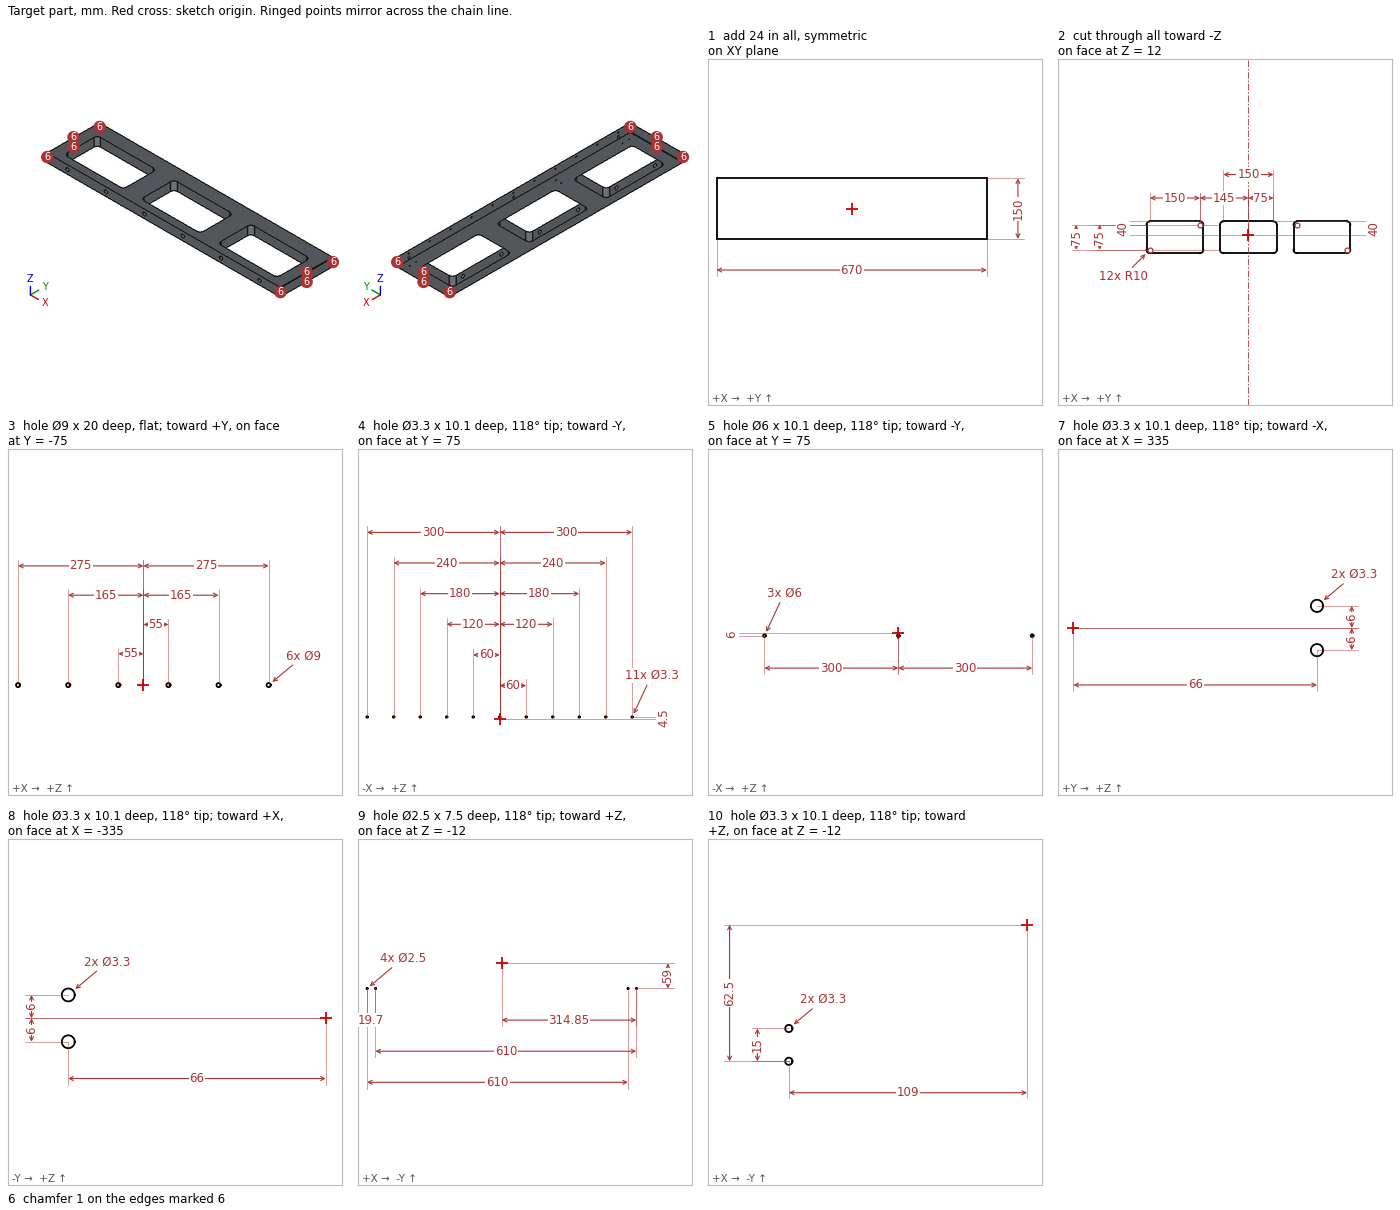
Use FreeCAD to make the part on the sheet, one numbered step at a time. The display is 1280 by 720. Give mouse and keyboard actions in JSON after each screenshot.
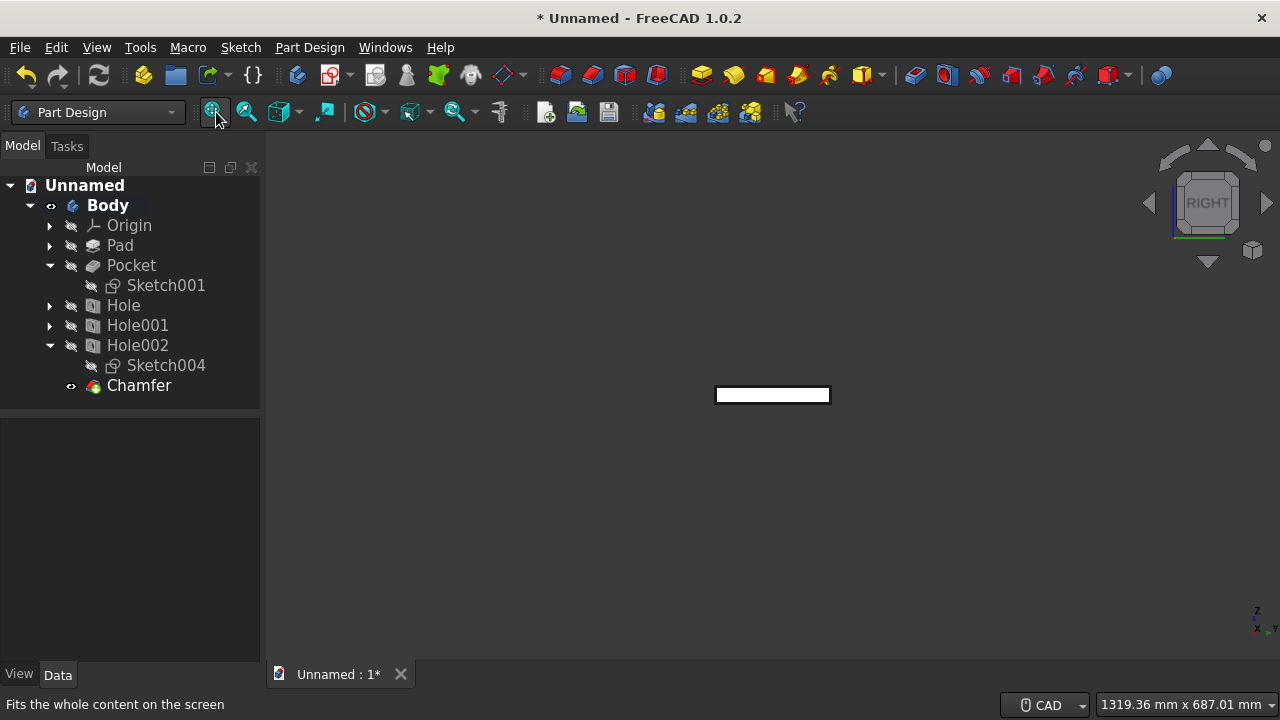
{"action": "left_click", "coordinate": [805, 394]}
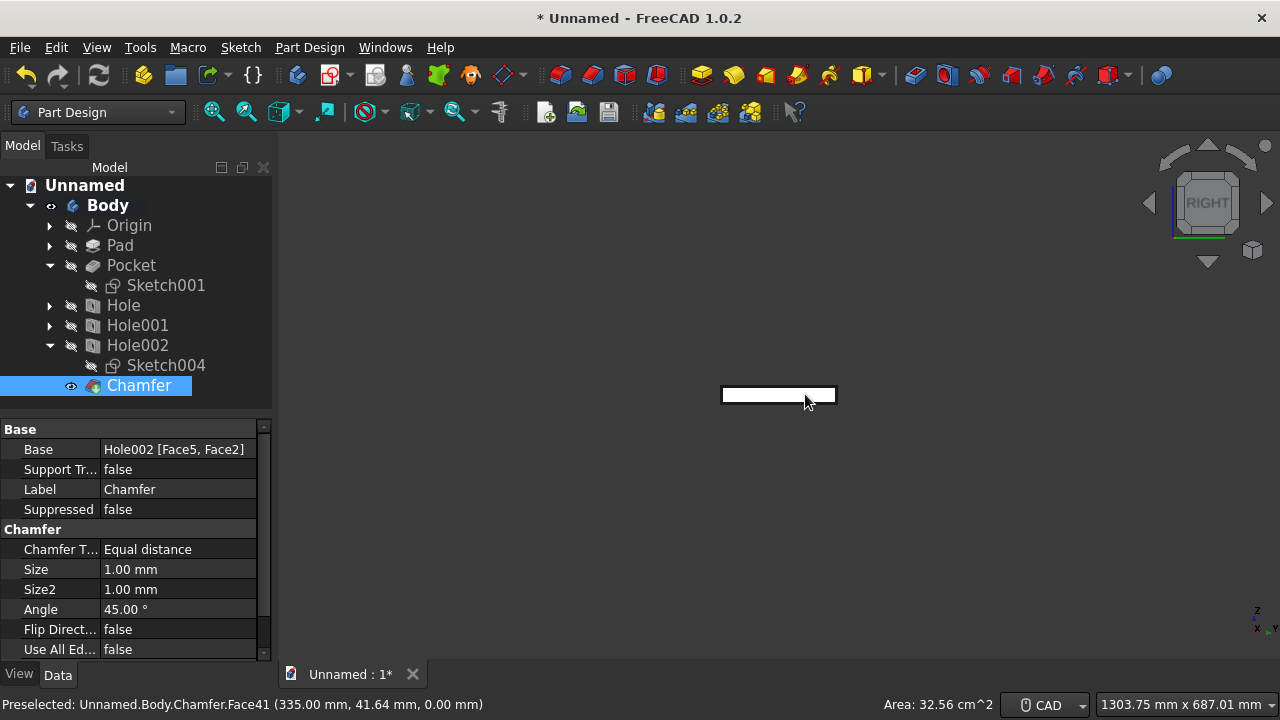
{"action": "left_click", "coordinate": [330, 76]}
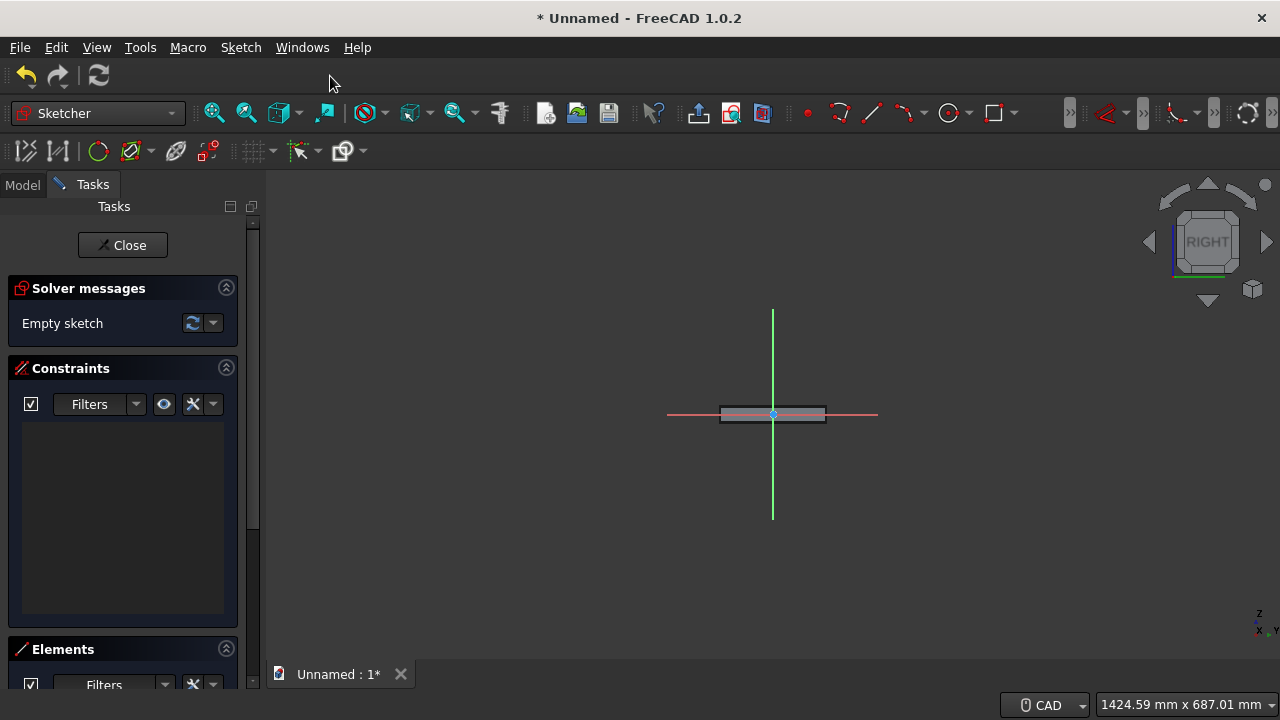
{"action": "scroll", "coordinate": [826, 414], "scroll_direction": "up", "scroll_amount": 15}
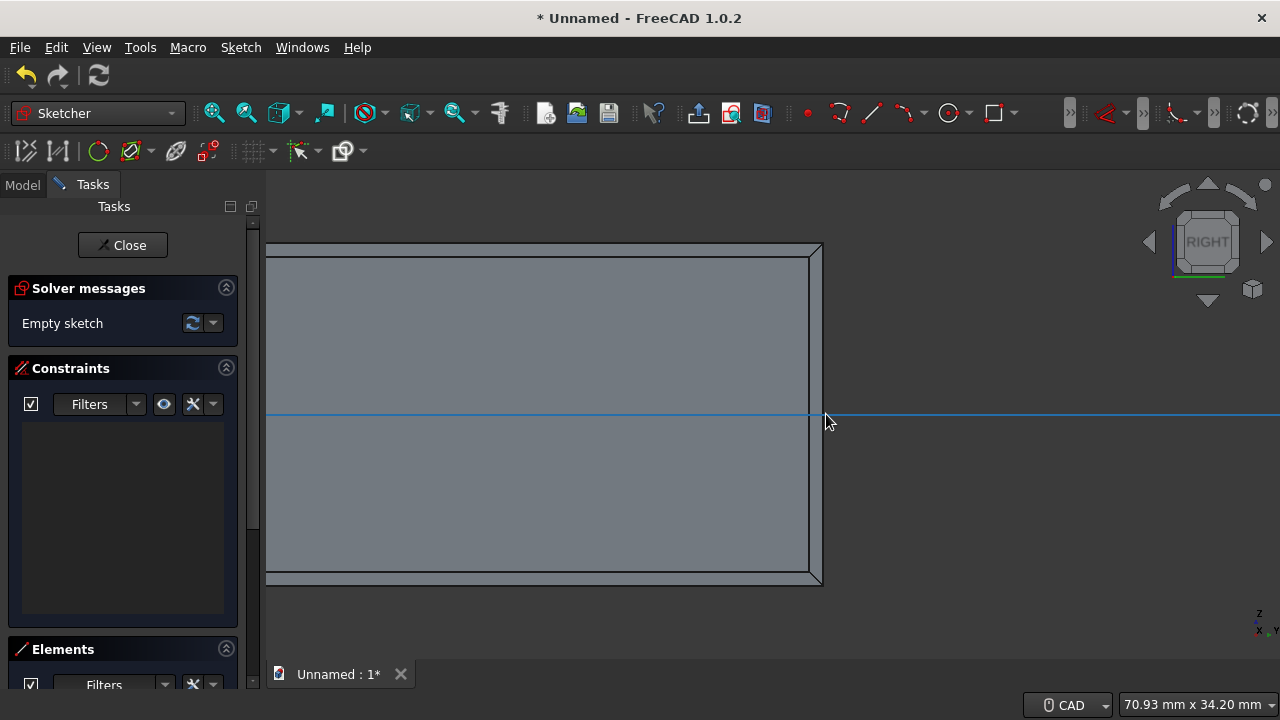
{"action": "scroll", "coordinate": [674, 414], "scroll_direction": "up", "scroll_amount": 2}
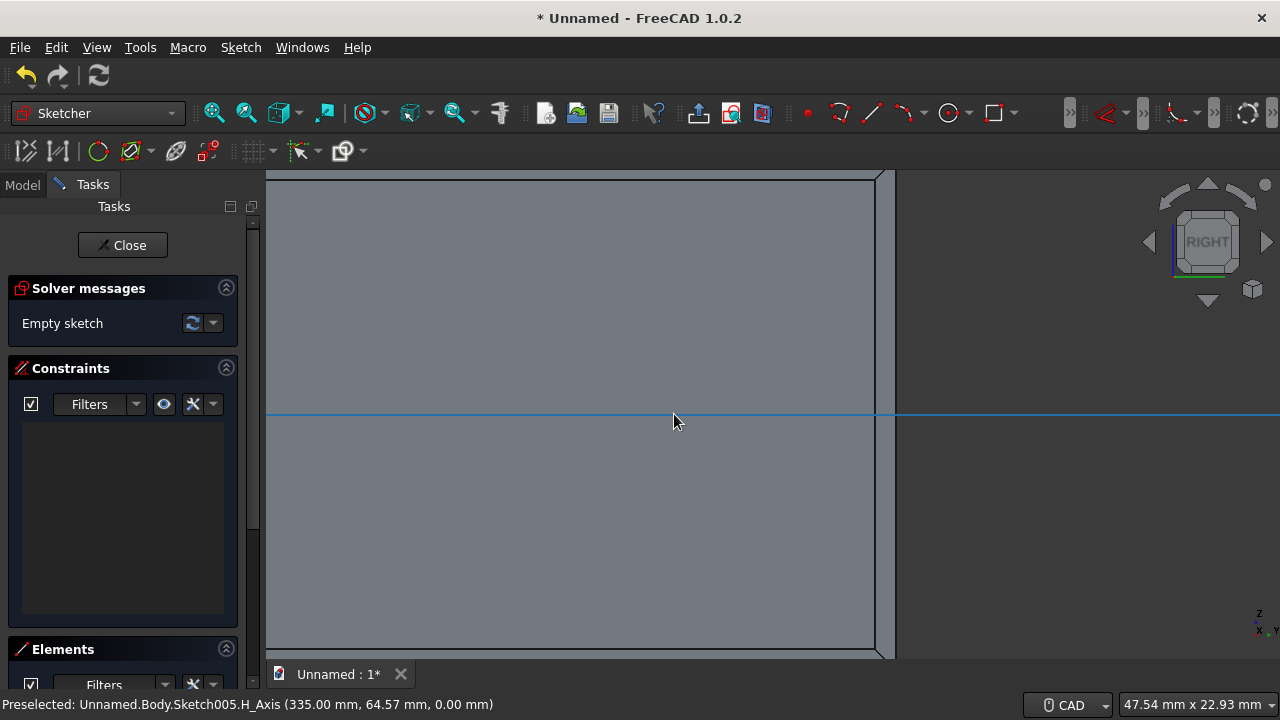
{"action": "left_click", "coordinate": [950, 114]}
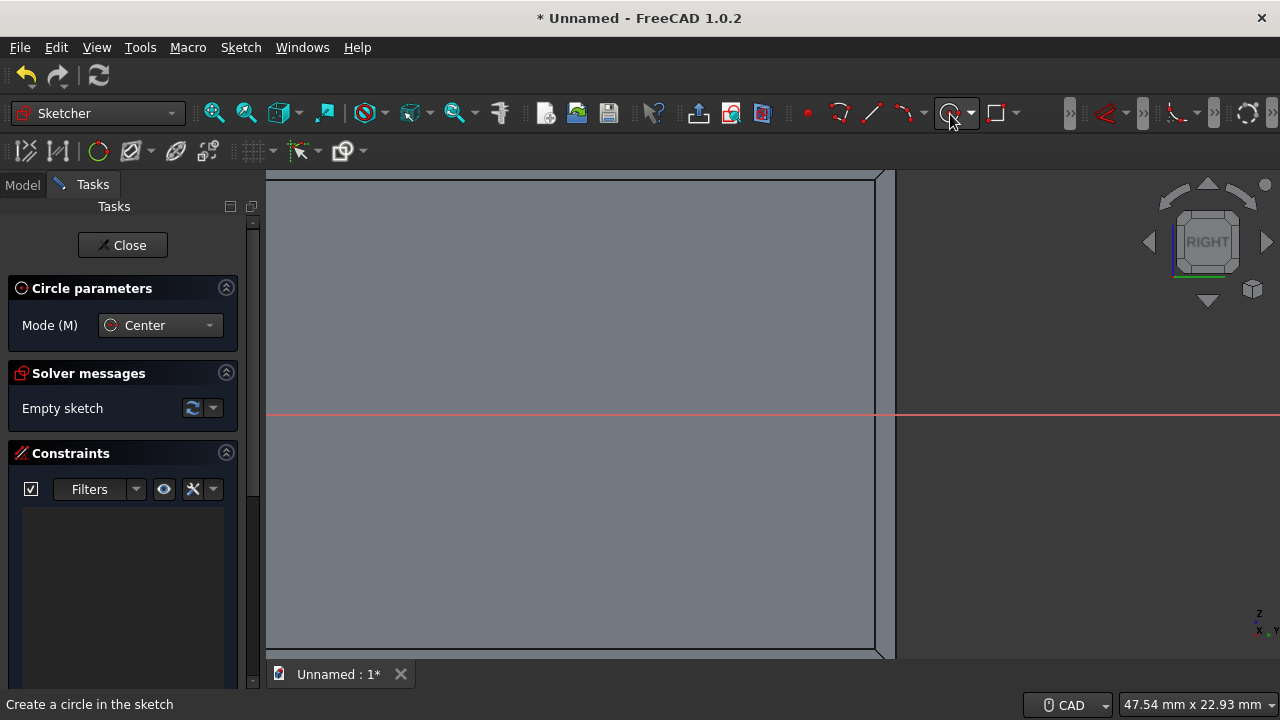
{"action": "left_click", "coordinate": [704, 542]}
{"action": "mouse_move", "coordinate": [729, 518]}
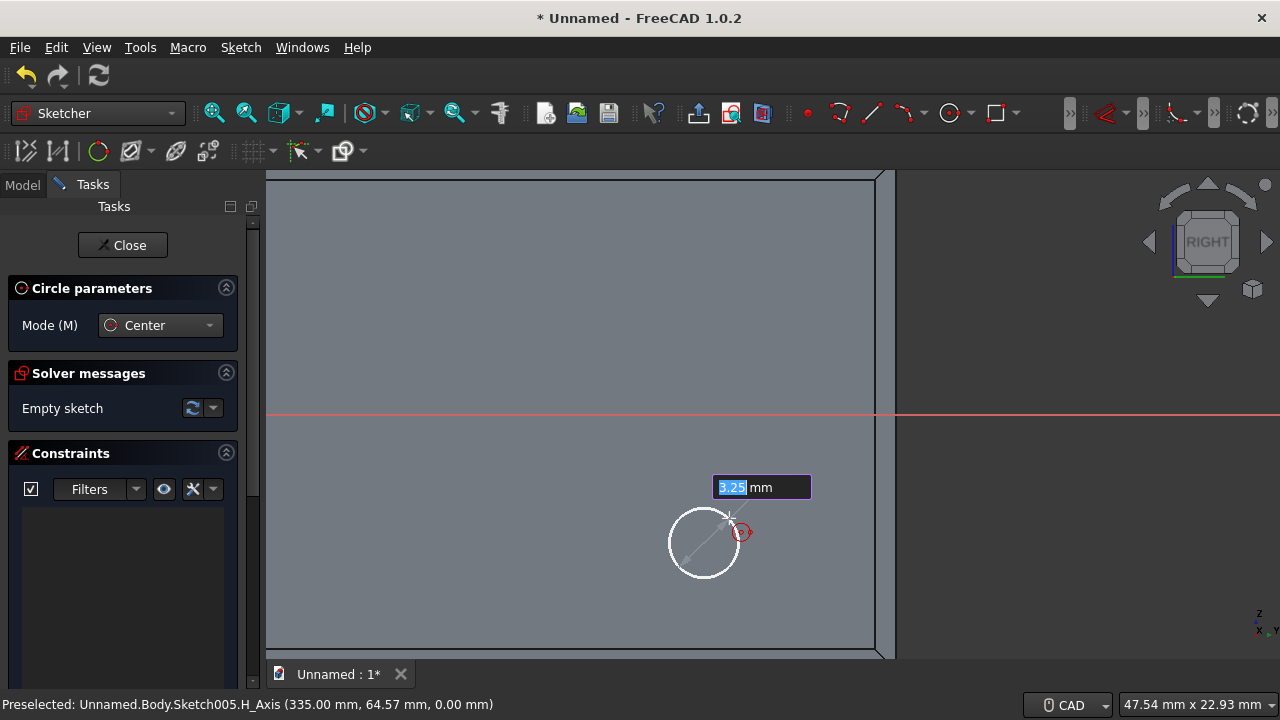
{"action": "type", "text": "3.3"}
{"action": "key", "text": "Return"}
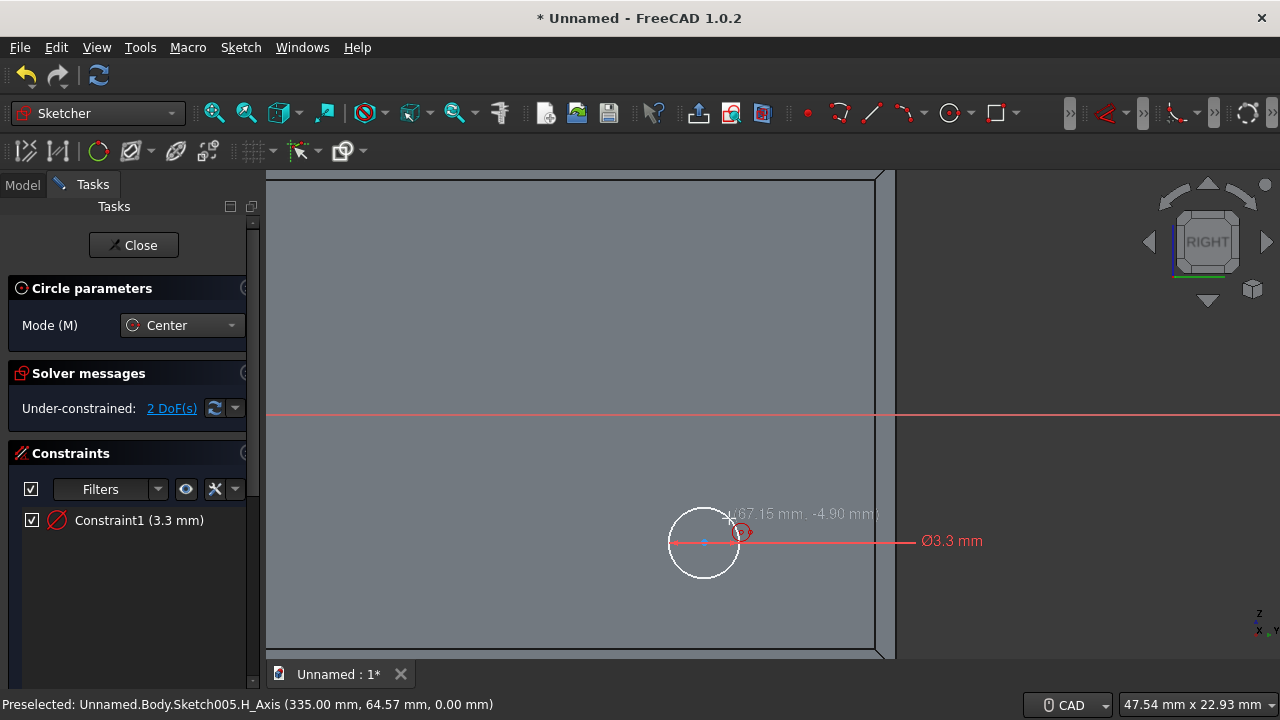
{"action": "left_click", "coordinate": [704, 287]}
{"action": "mouse_move", "coordinate": [729, 262]}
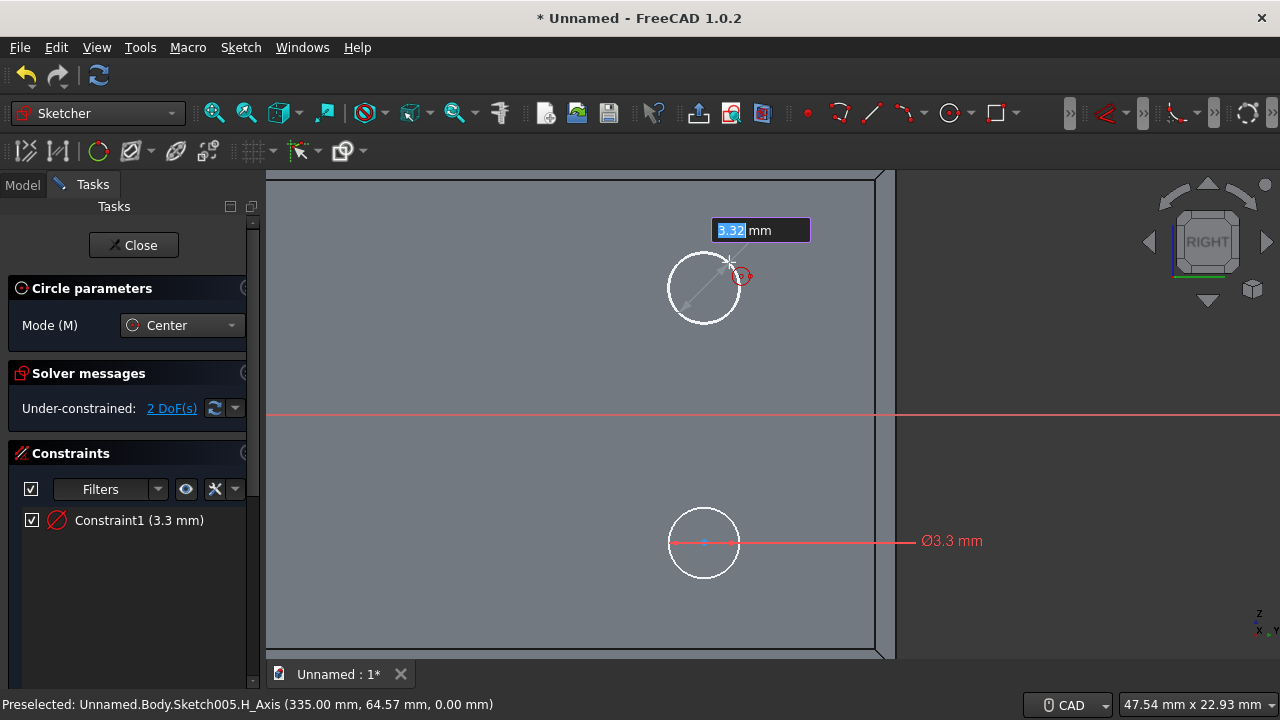
{"action": "type", "text": "3.3"}
{"action": "key", "text": "Return"}
{"action": "key", "text": "Escape"}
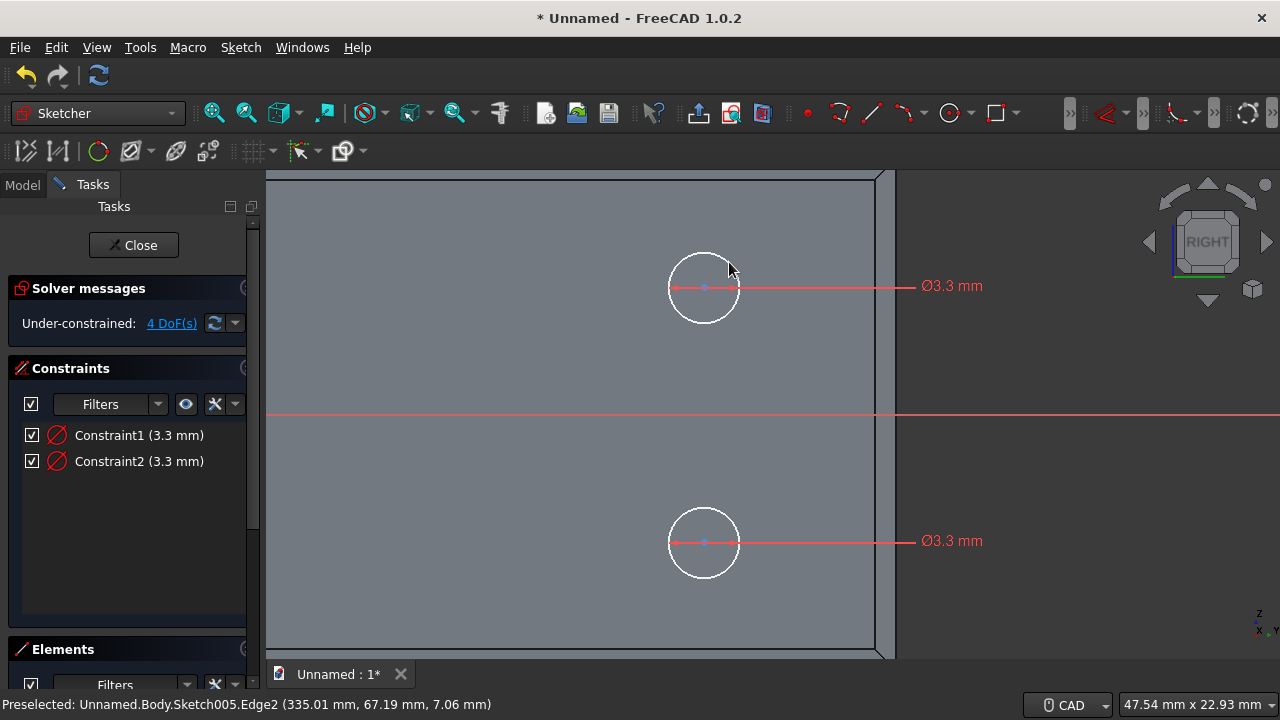
{"action": "left_click", "coordinate": [704, 543]}